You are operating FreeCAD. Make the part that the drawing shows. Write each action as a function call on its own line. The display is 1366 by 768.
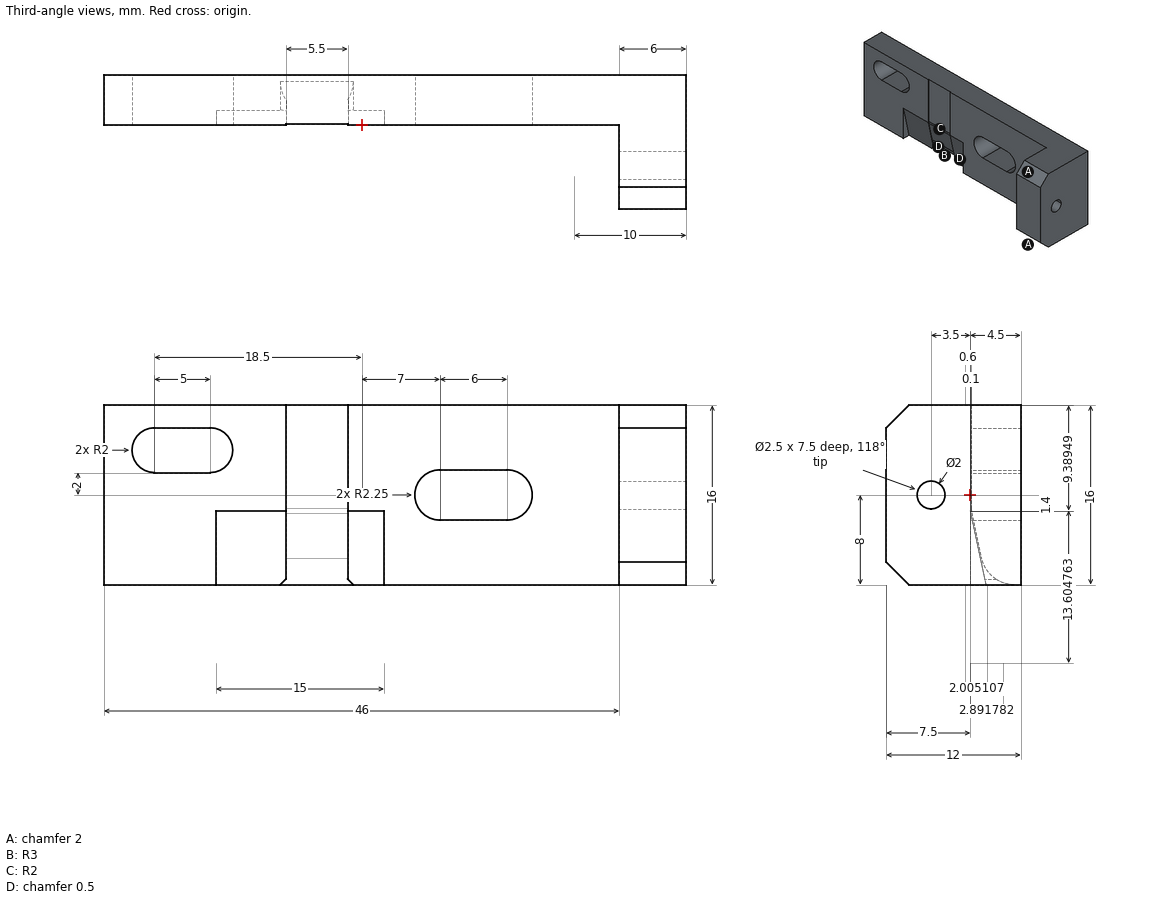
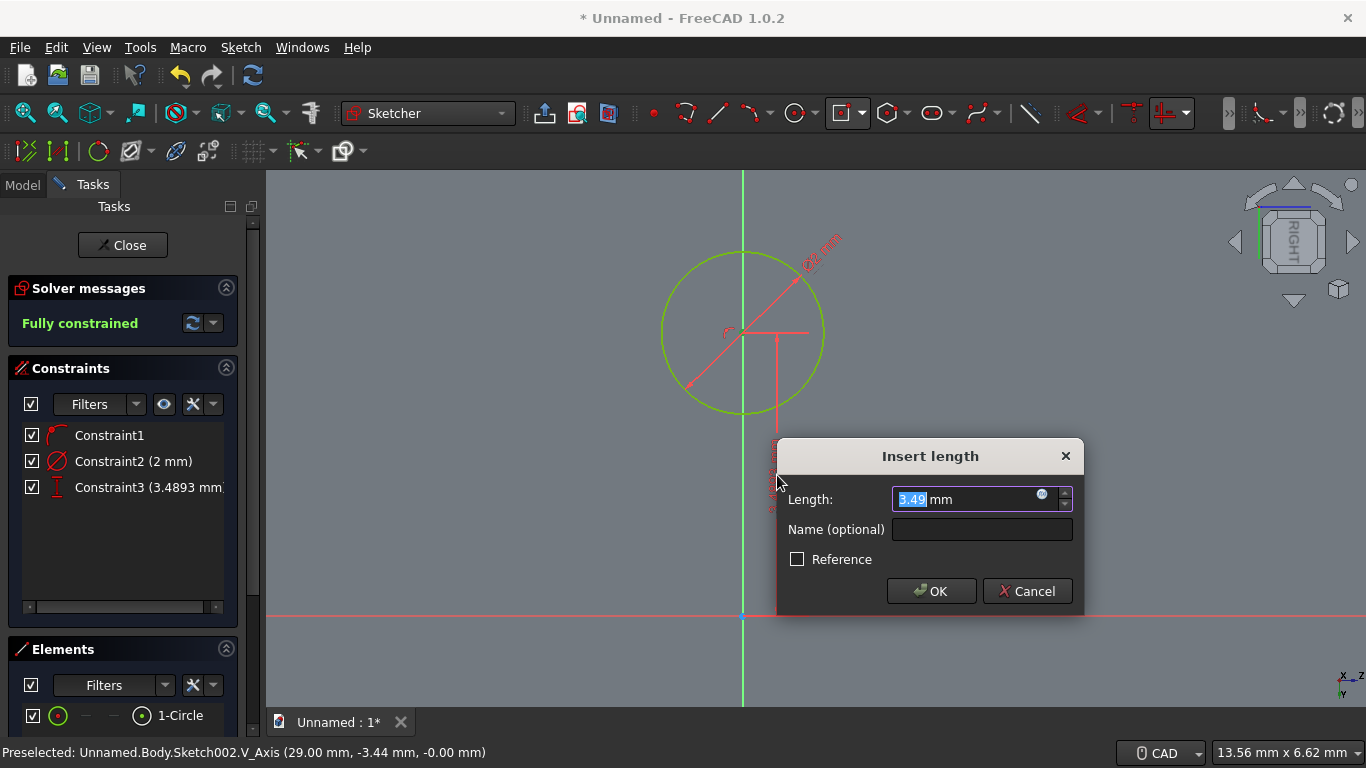
text(3.5)
key(Return)
key(Escape)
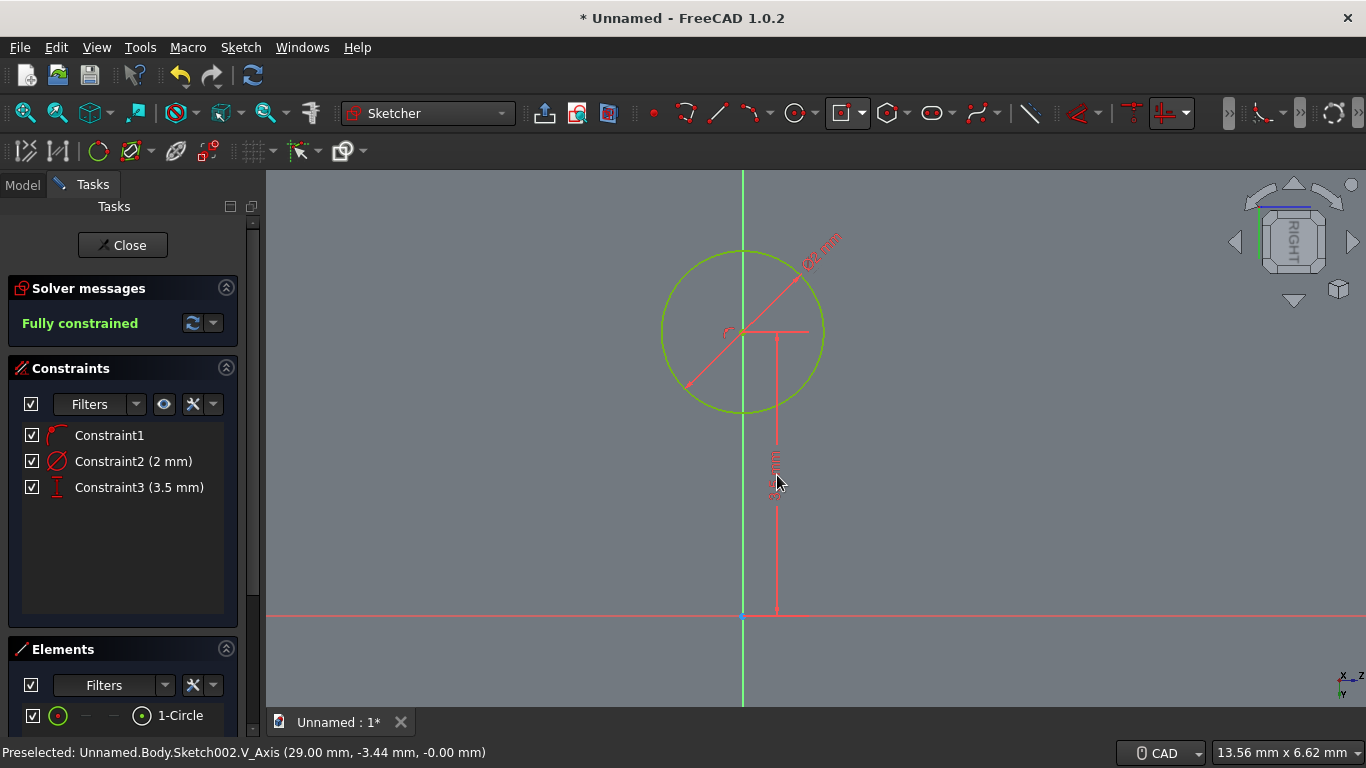
click(123, 245)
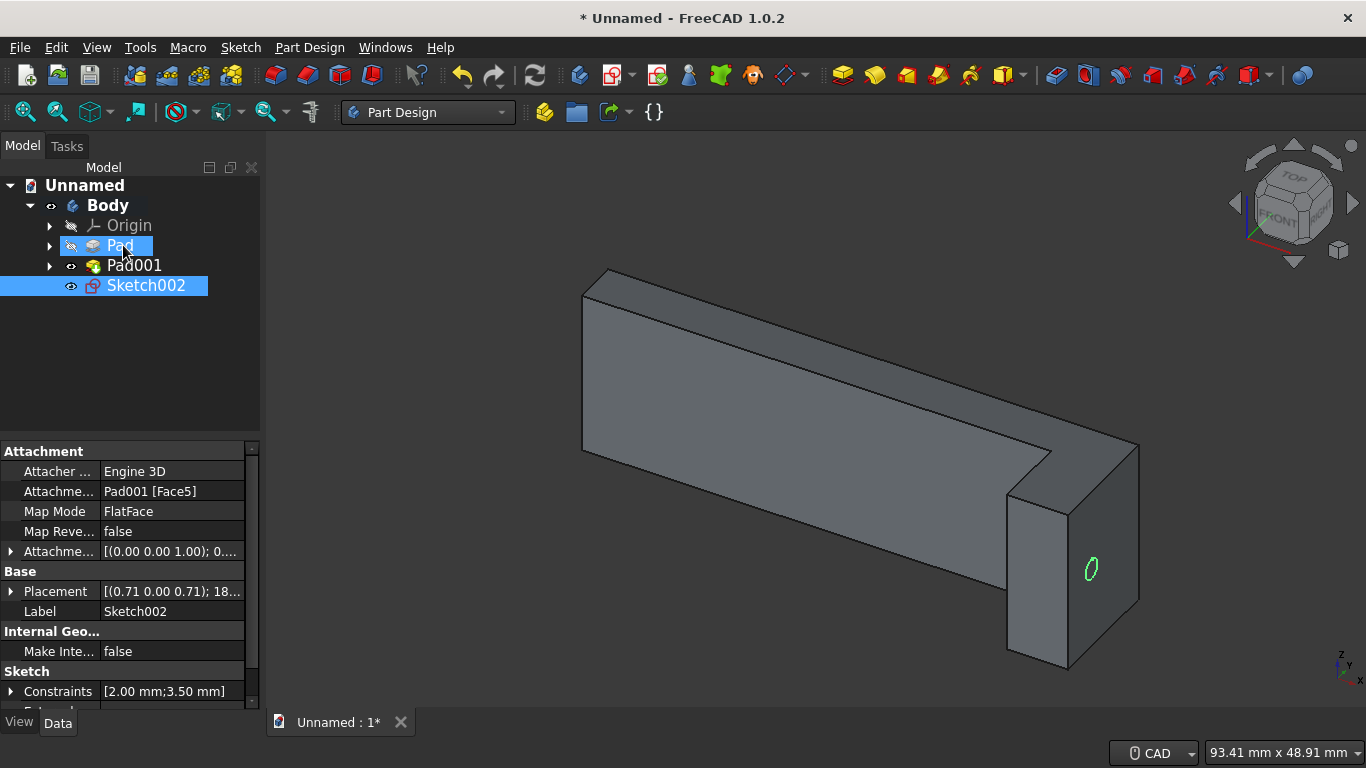
click(1058, 76)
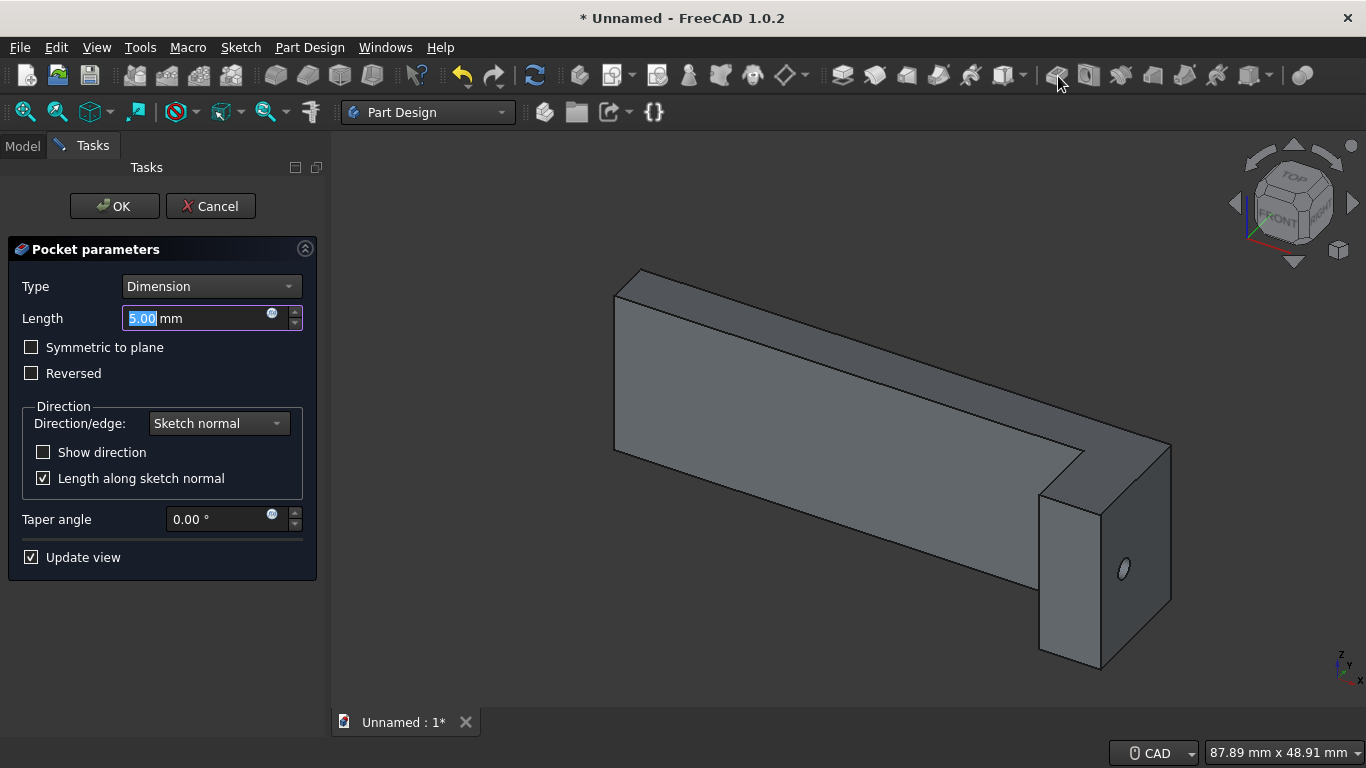
text(10)
key(Tab)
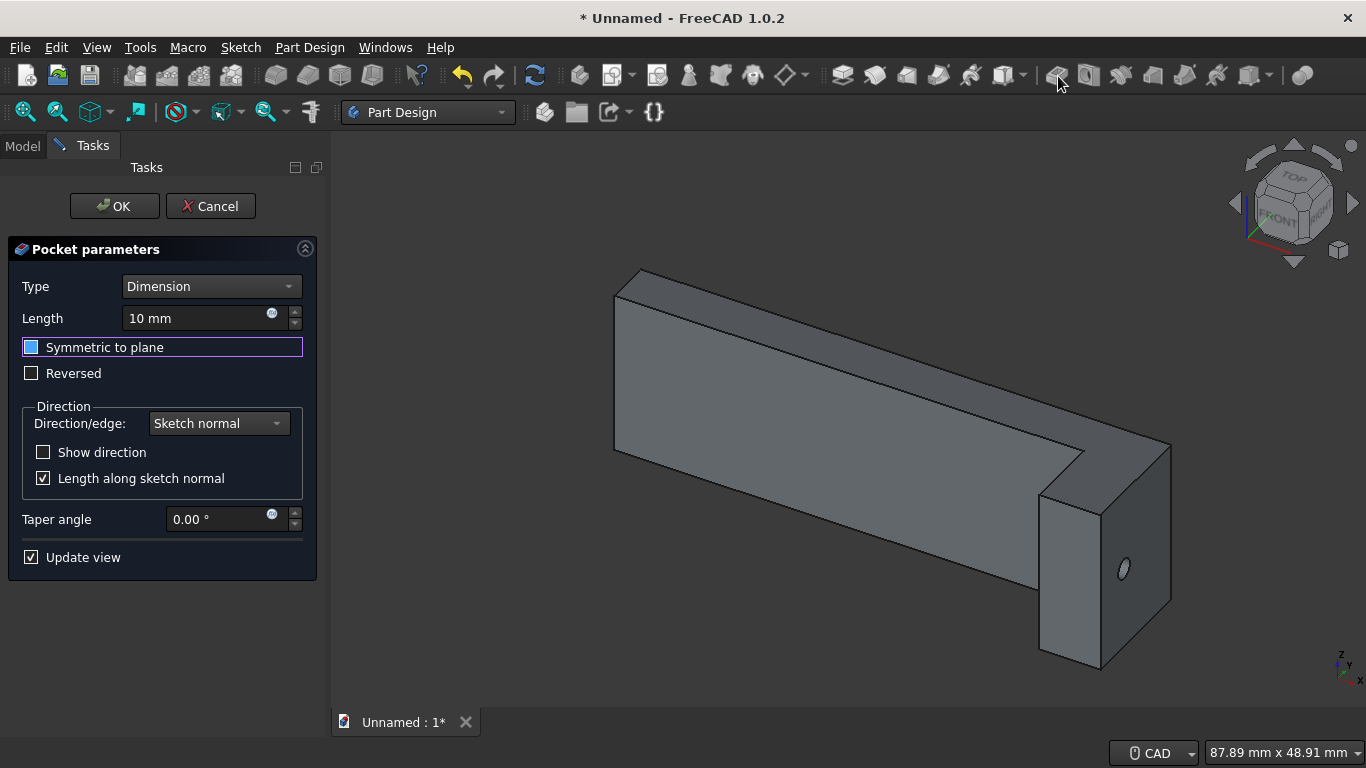
click(115, 206)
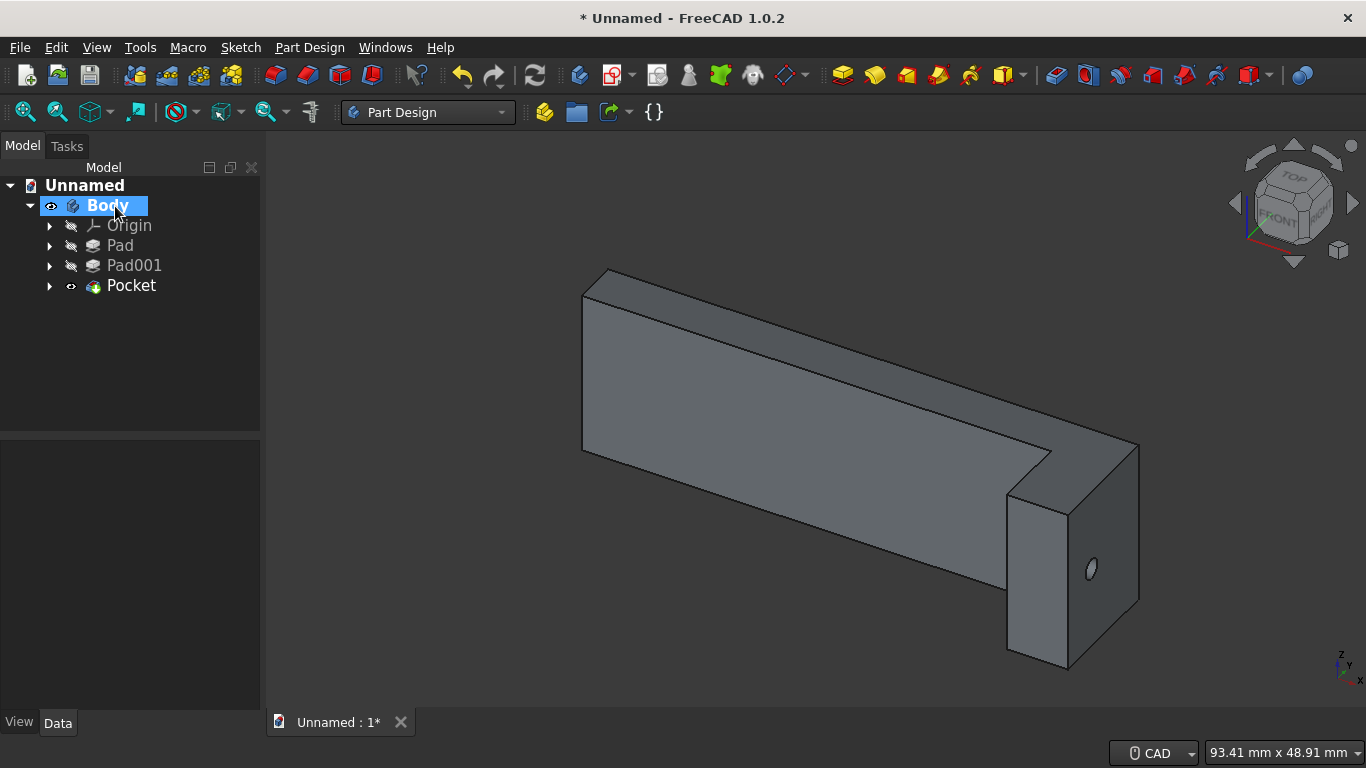
click(1113, 502)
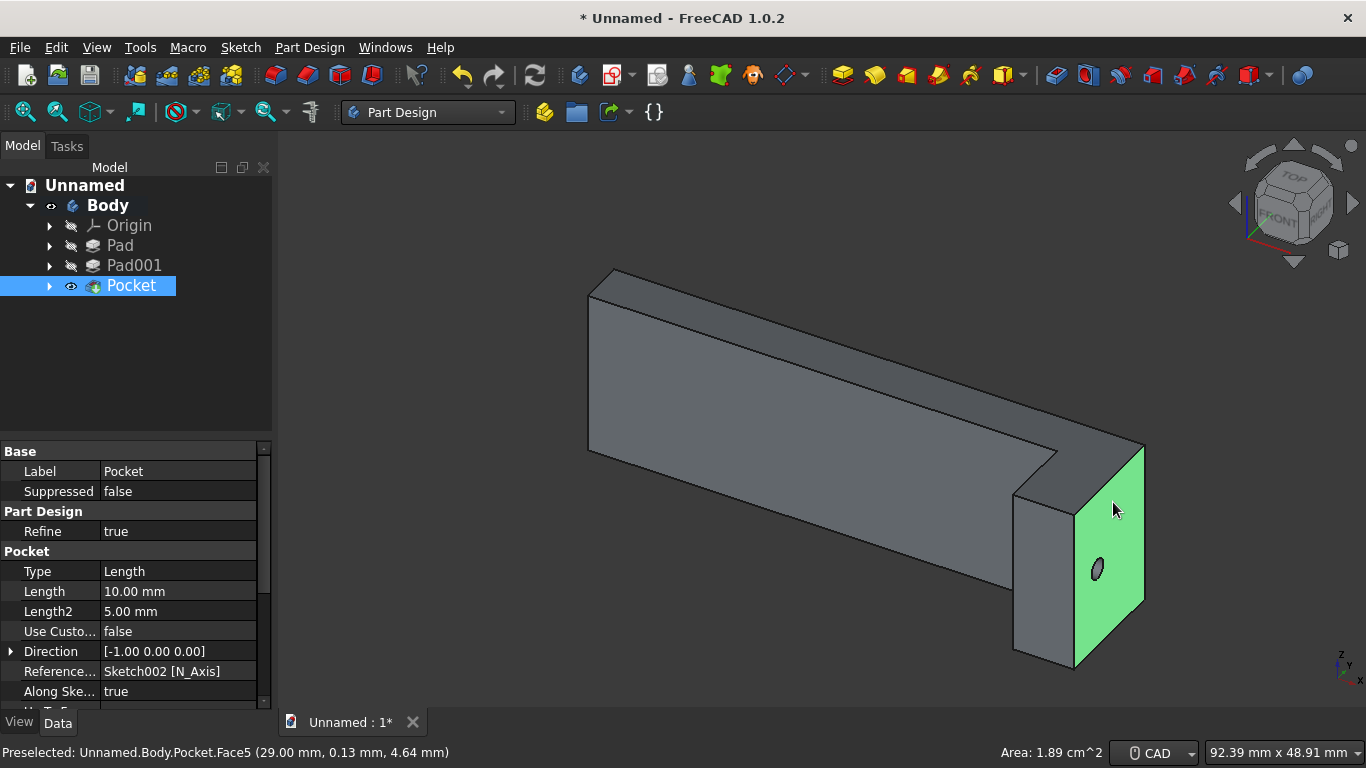
click(612, 76)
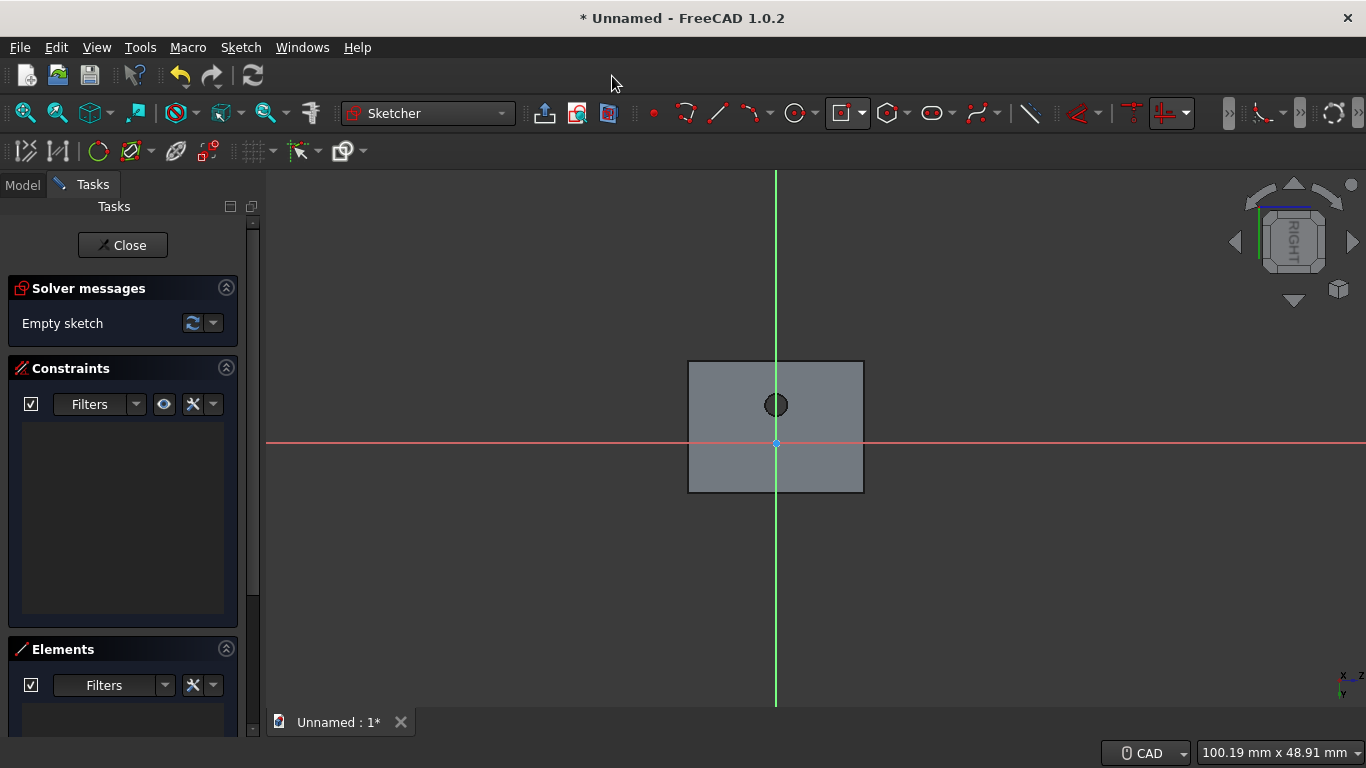
scroll(782, 413, up, 9)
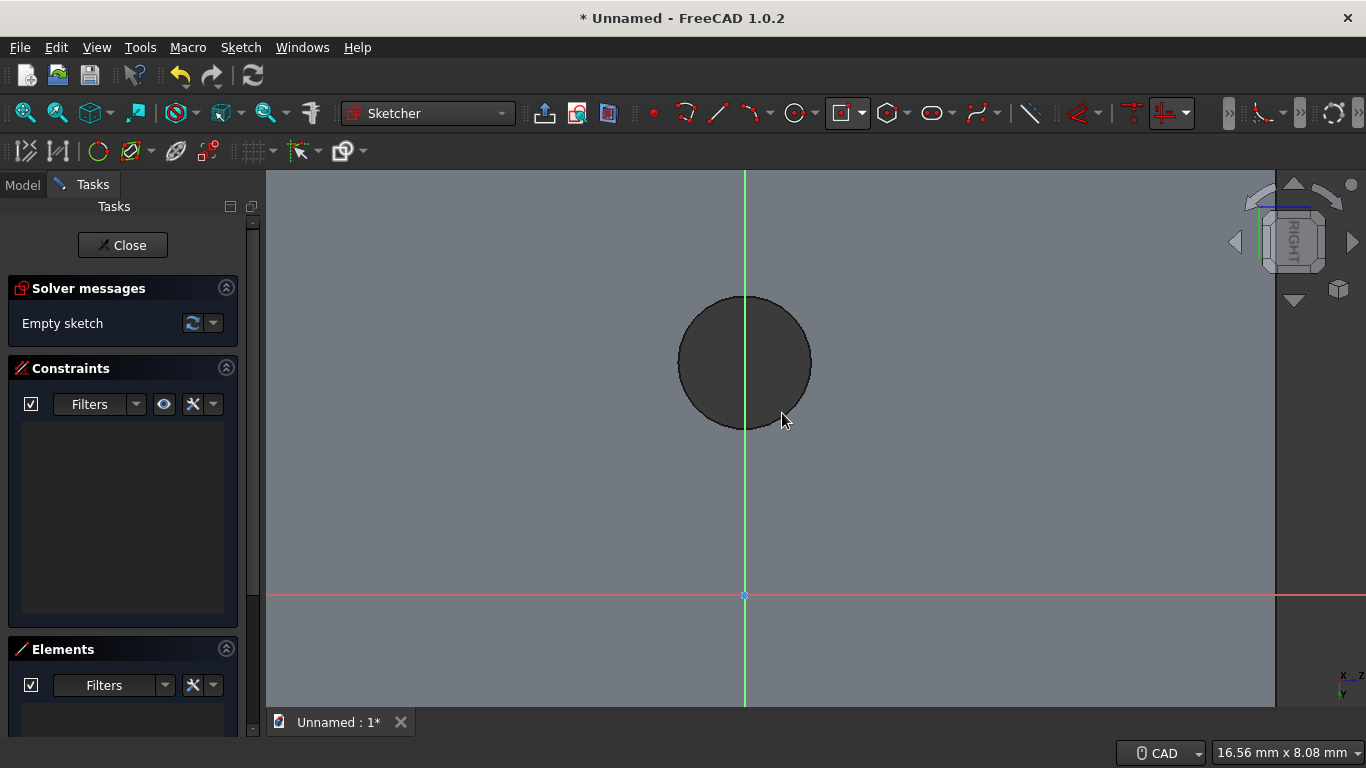
key(g)
key(c)